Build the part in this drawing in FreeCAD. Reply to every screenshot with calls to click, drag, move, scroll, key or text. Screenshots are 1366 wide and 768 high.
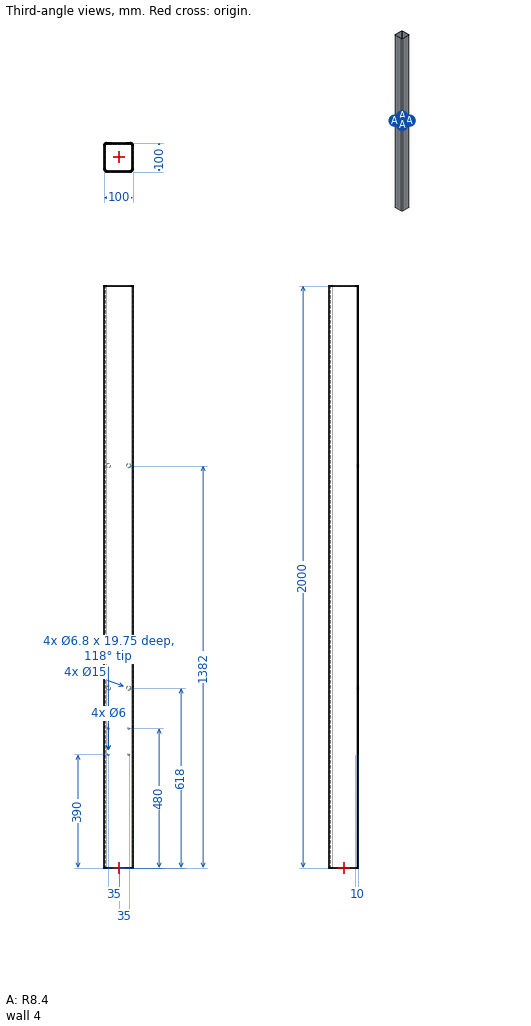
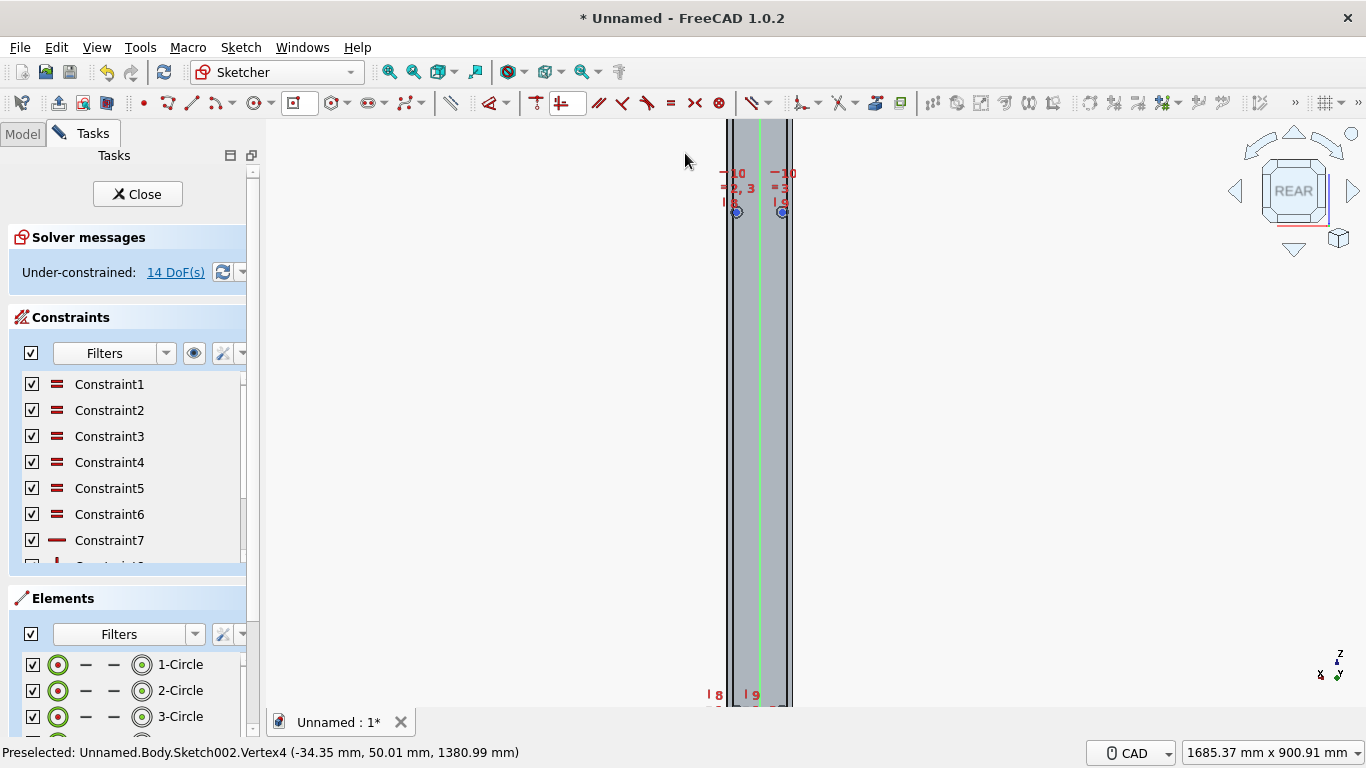
scroll(737, 212, down, 4)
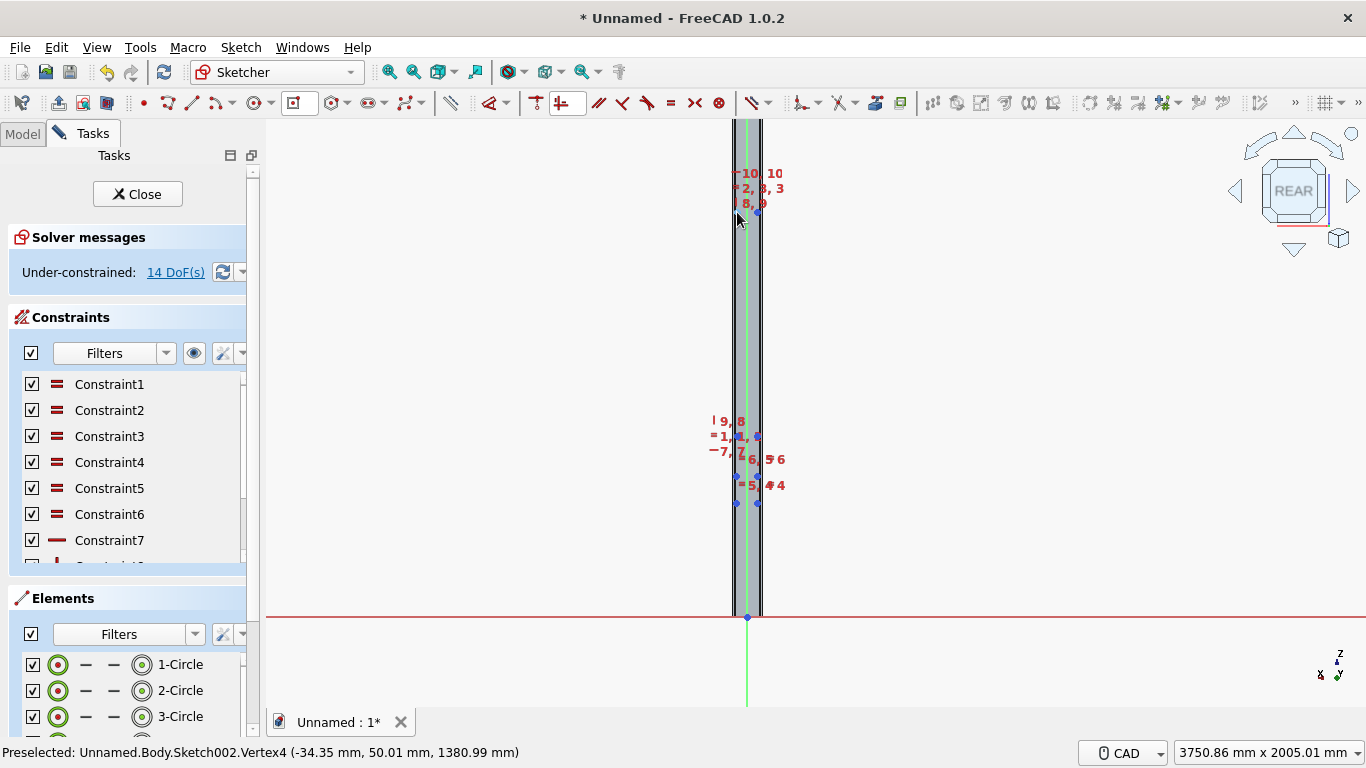
click(758, 436)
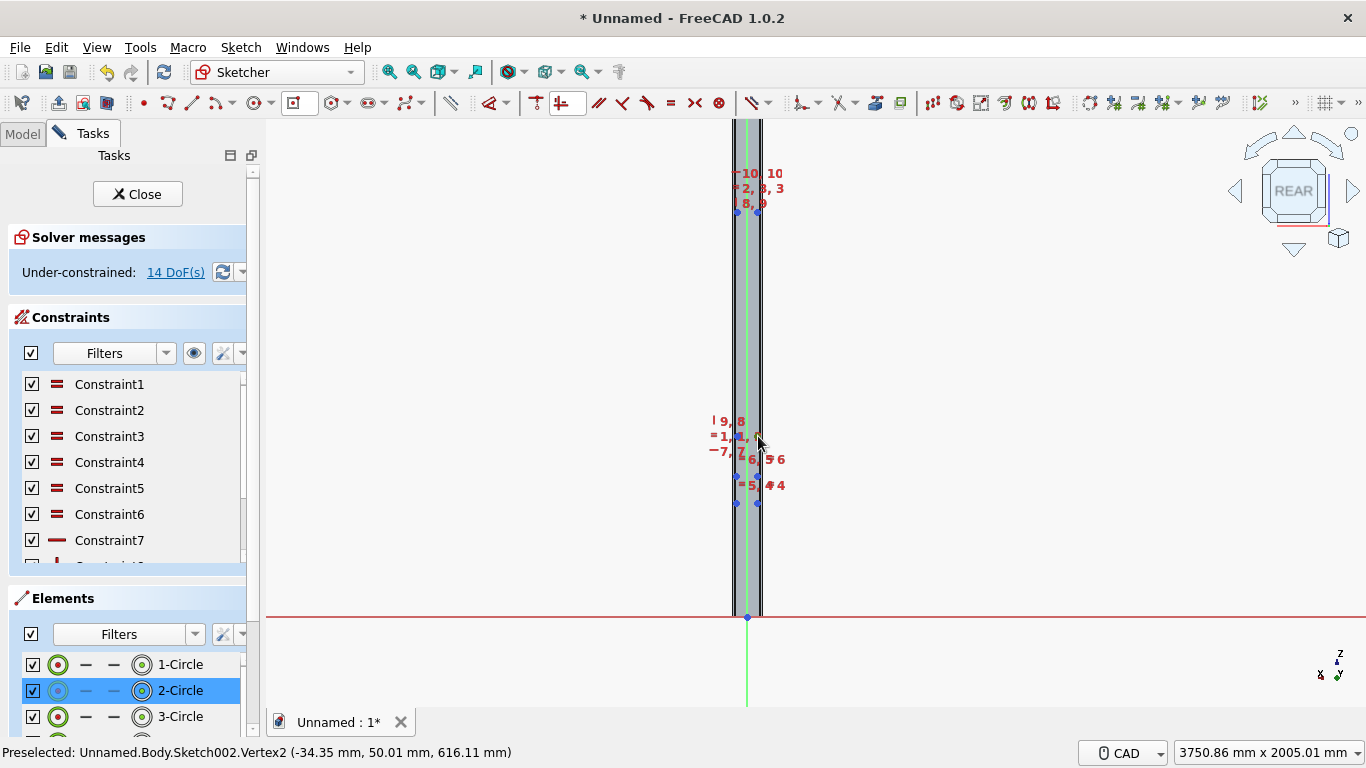
click(758, 503)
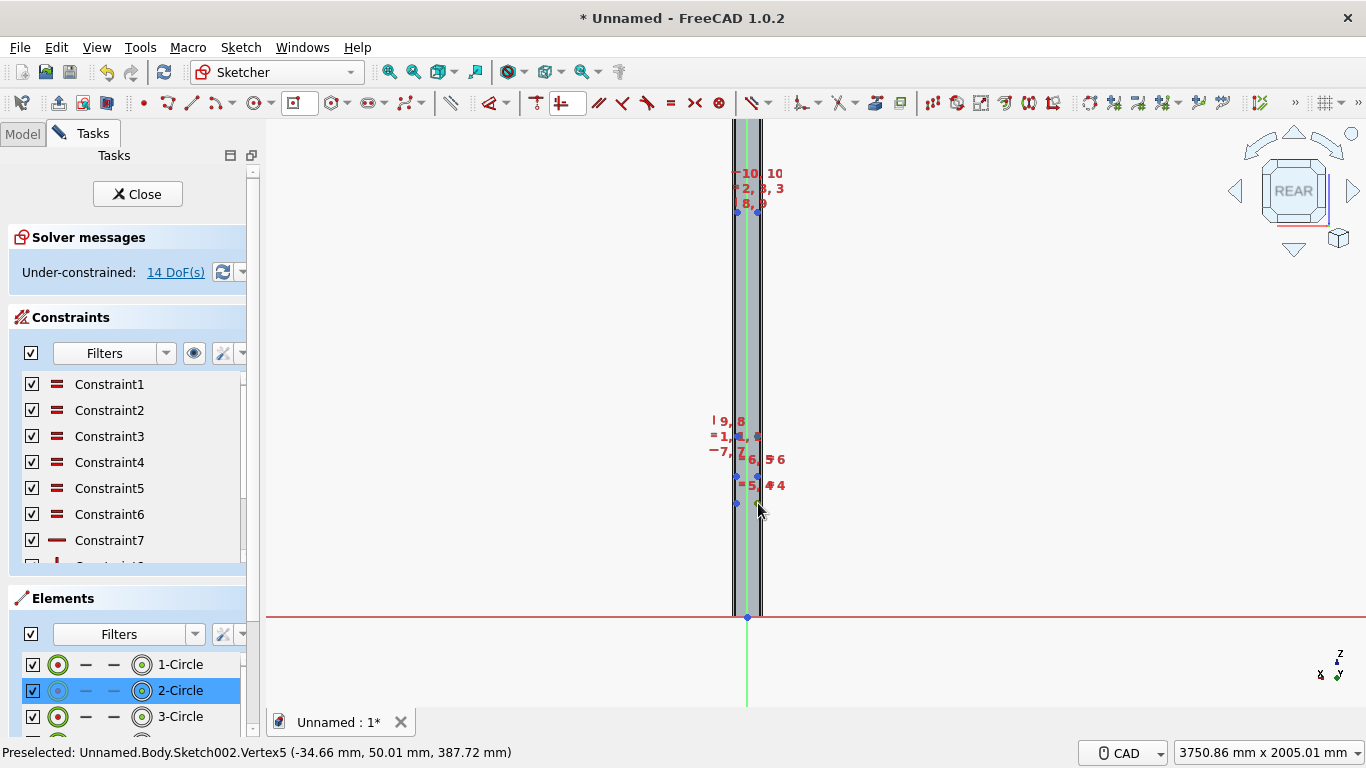
key(v)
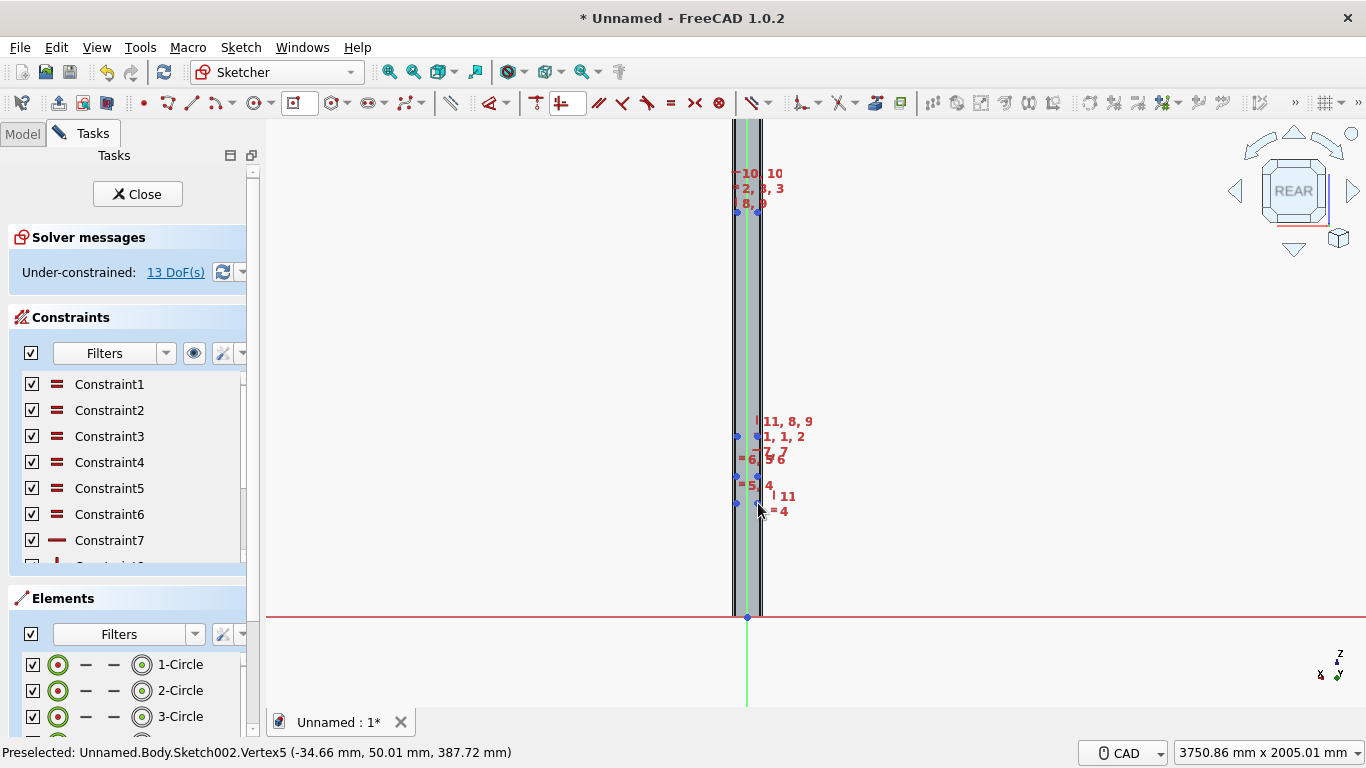
click(737, 436)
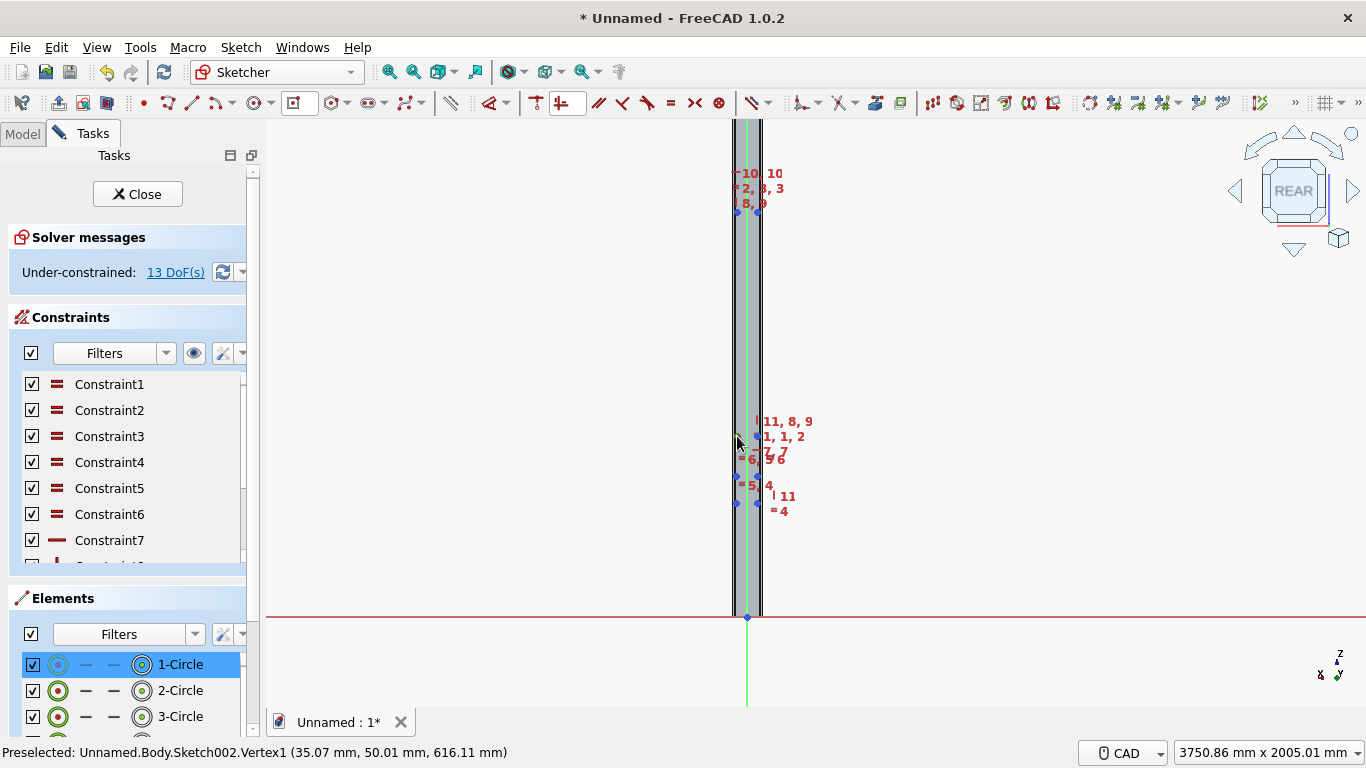
click(737, 503)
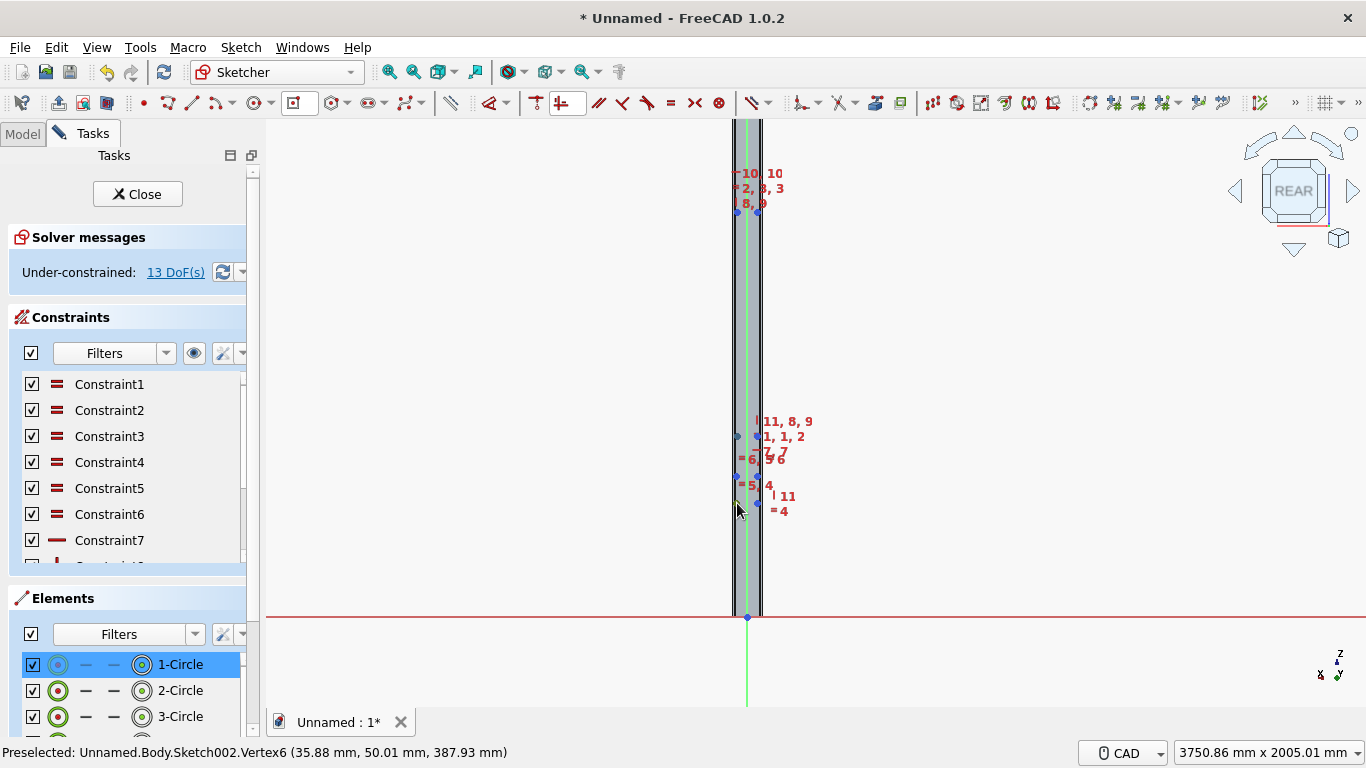
key(v)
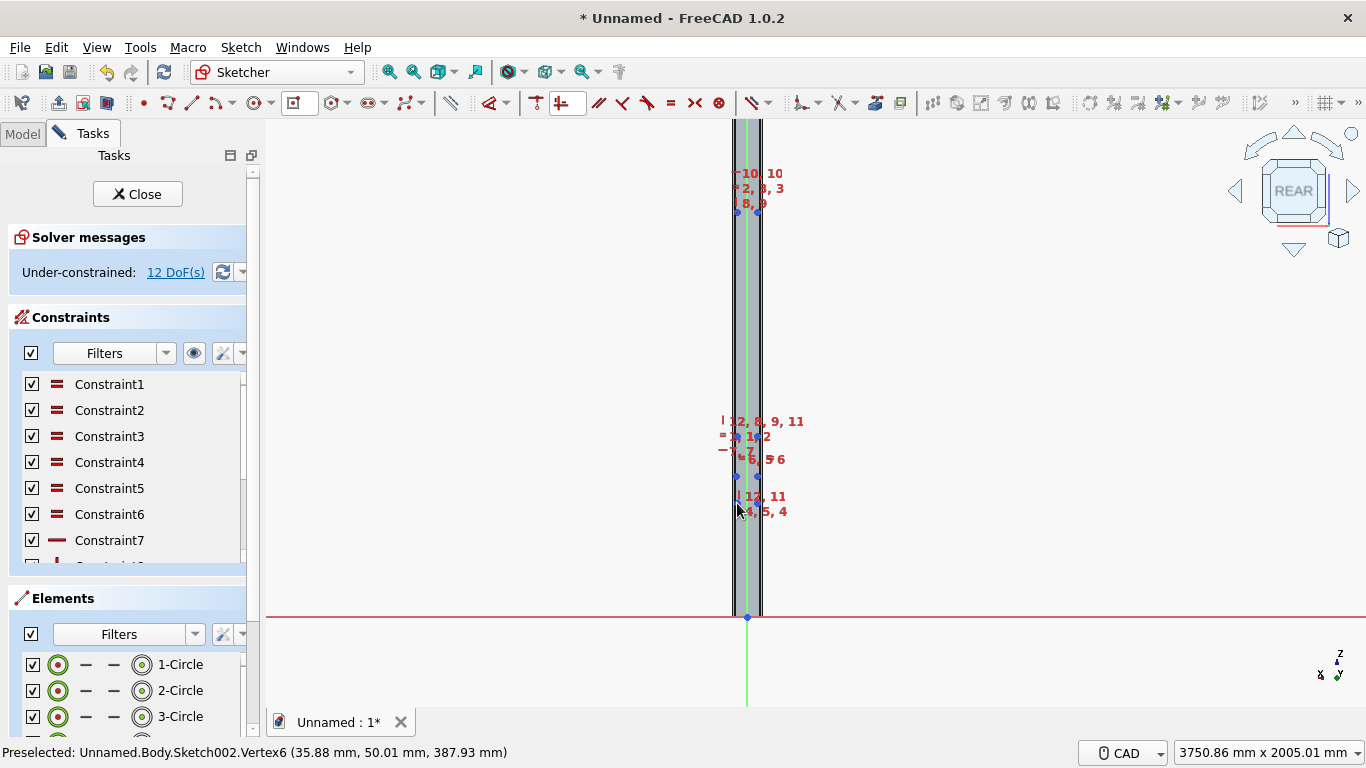
scroll(758, 503, up, 4)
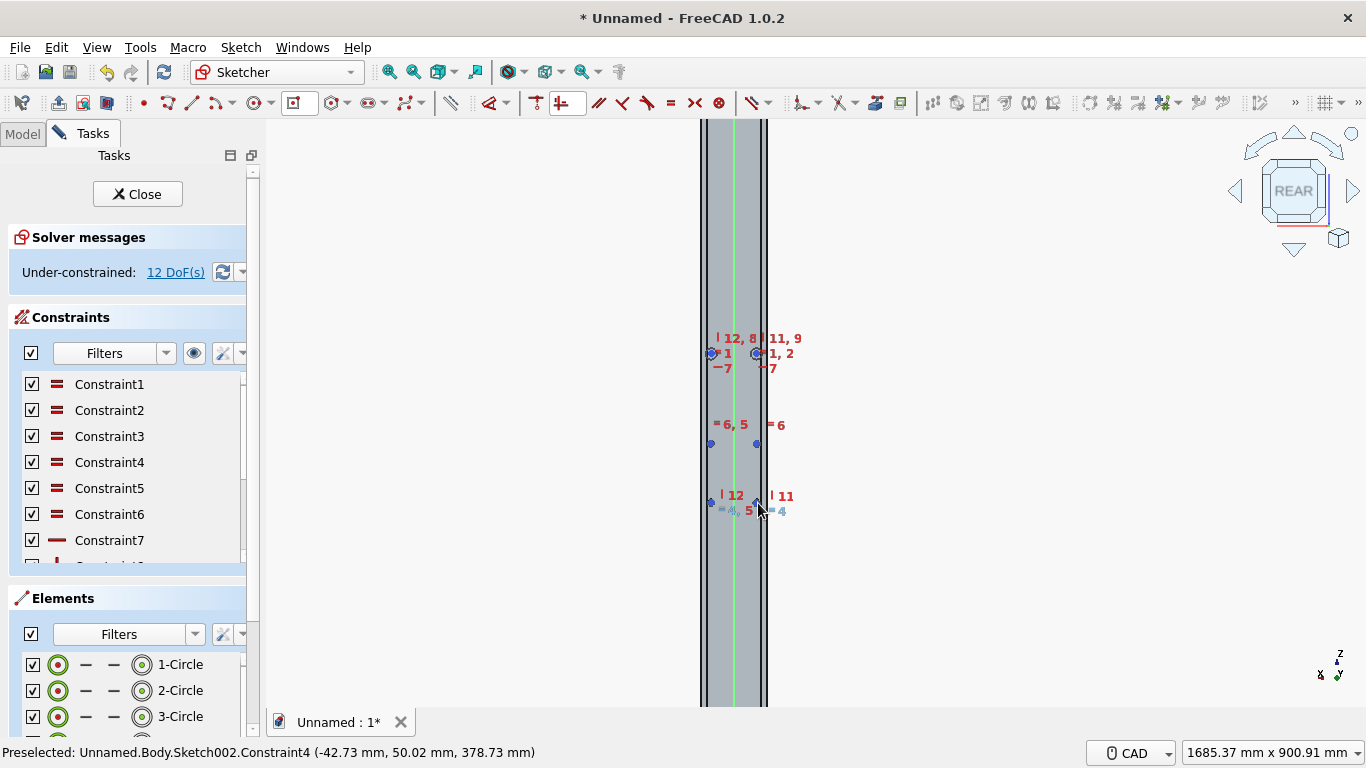
click(756, 503)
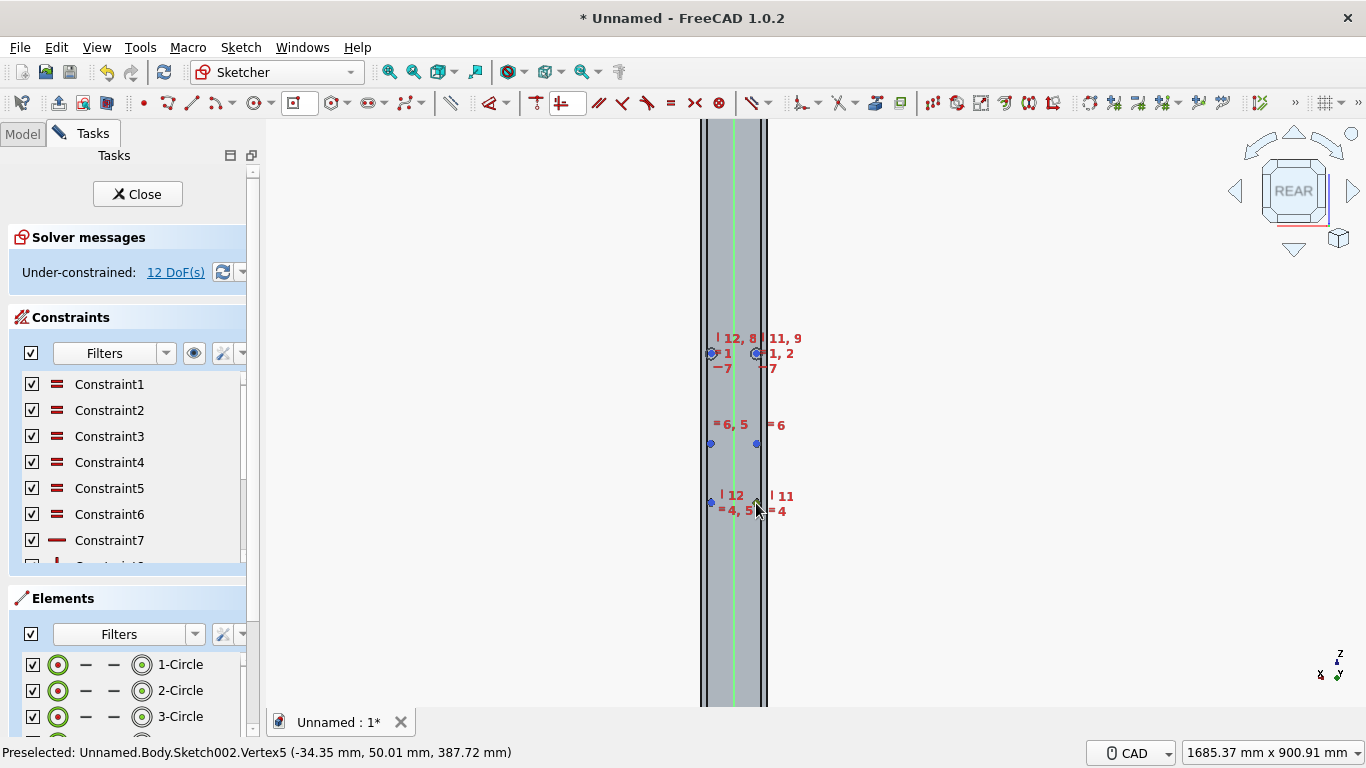
click(711, 503)